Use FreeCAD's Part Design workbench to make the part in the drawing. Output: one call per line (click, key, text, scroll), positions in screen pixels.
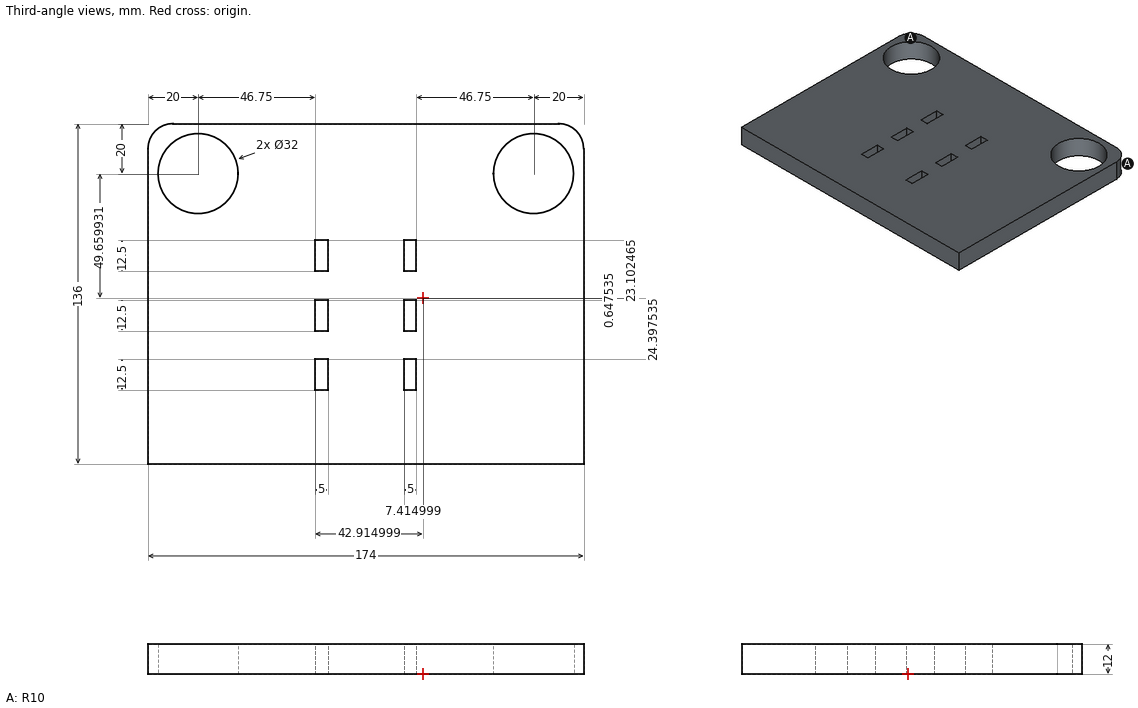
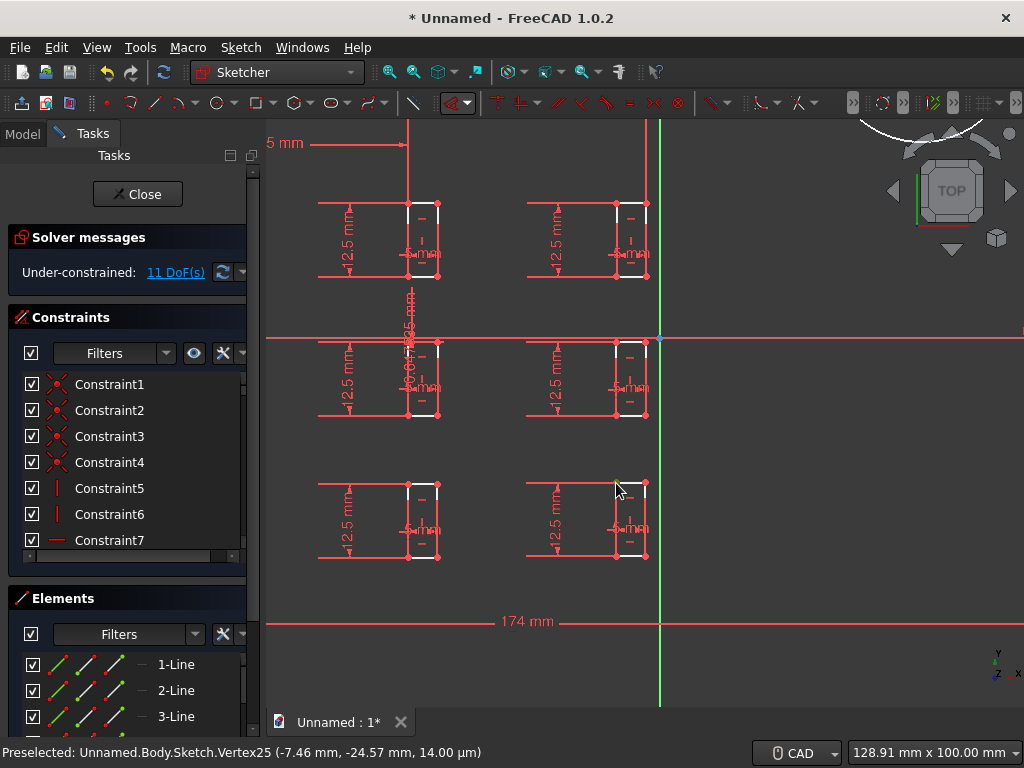
key(l)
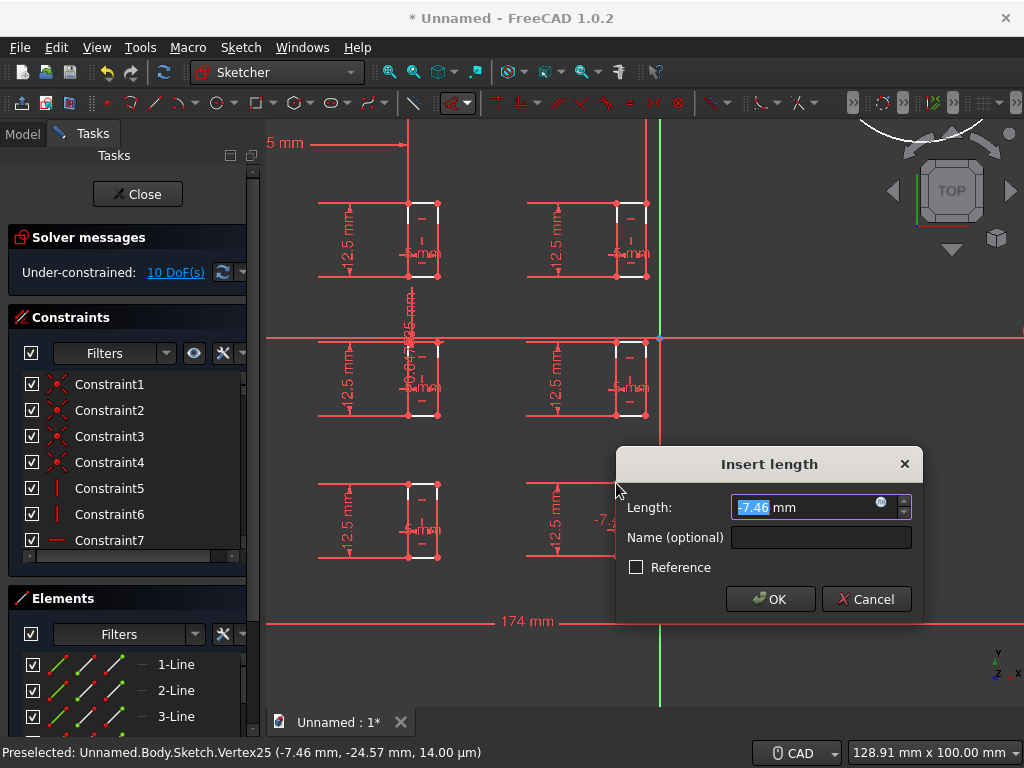
text(-7.414999)
key(Return)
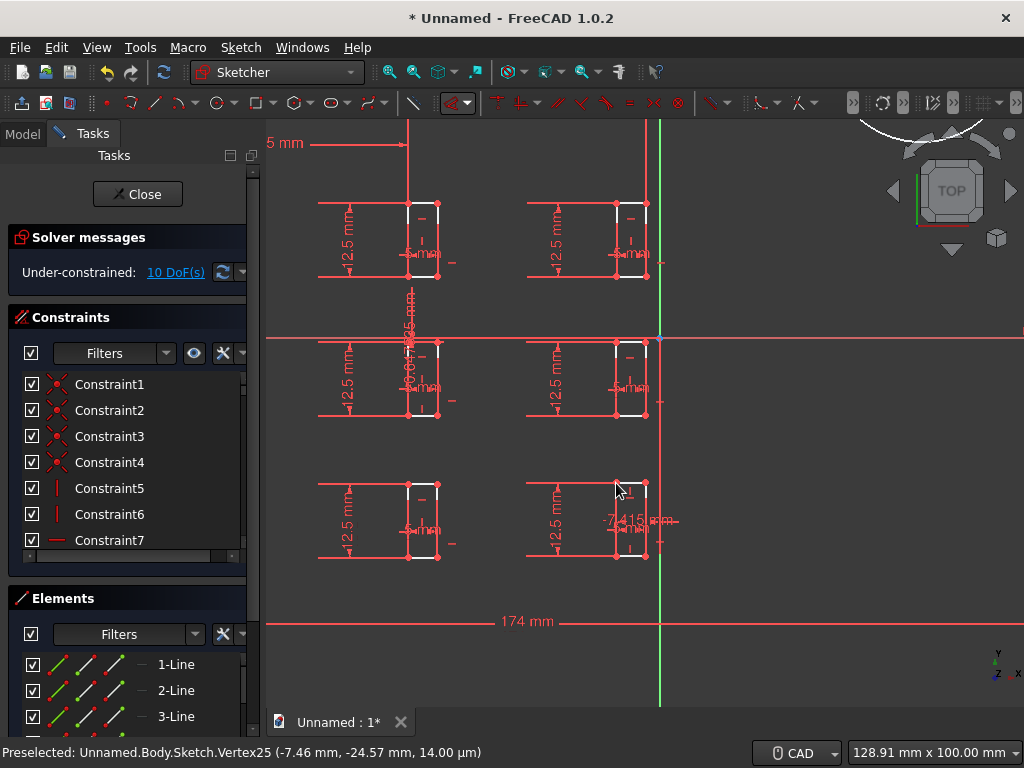
click(616, 342)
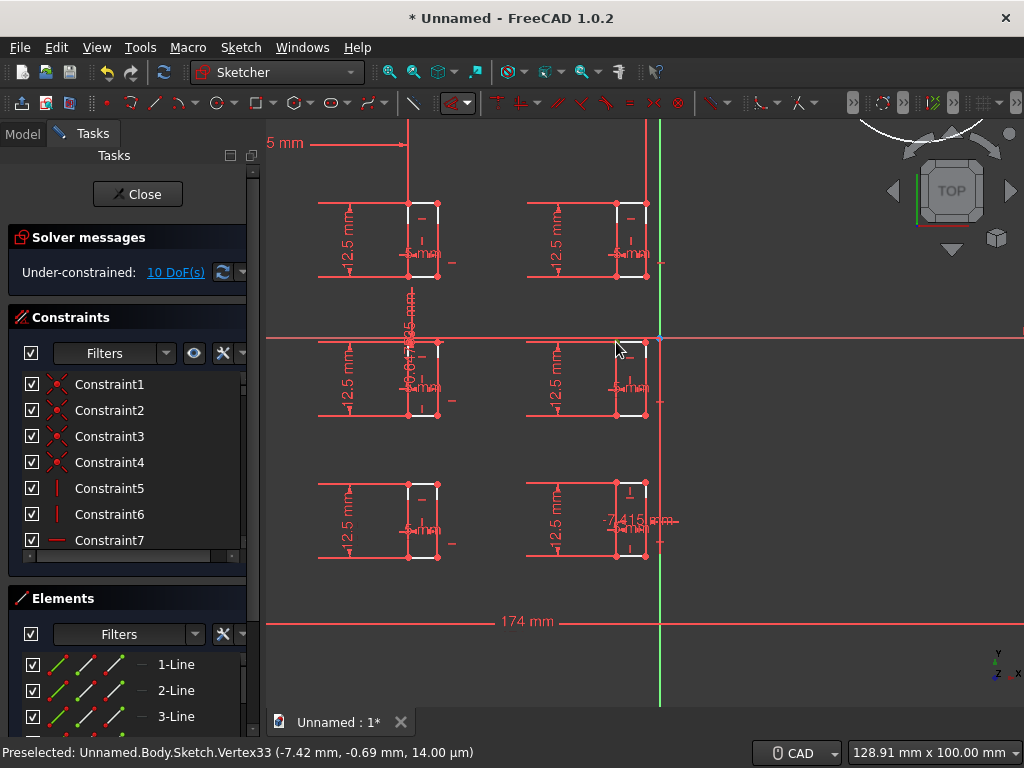
click(470, 104)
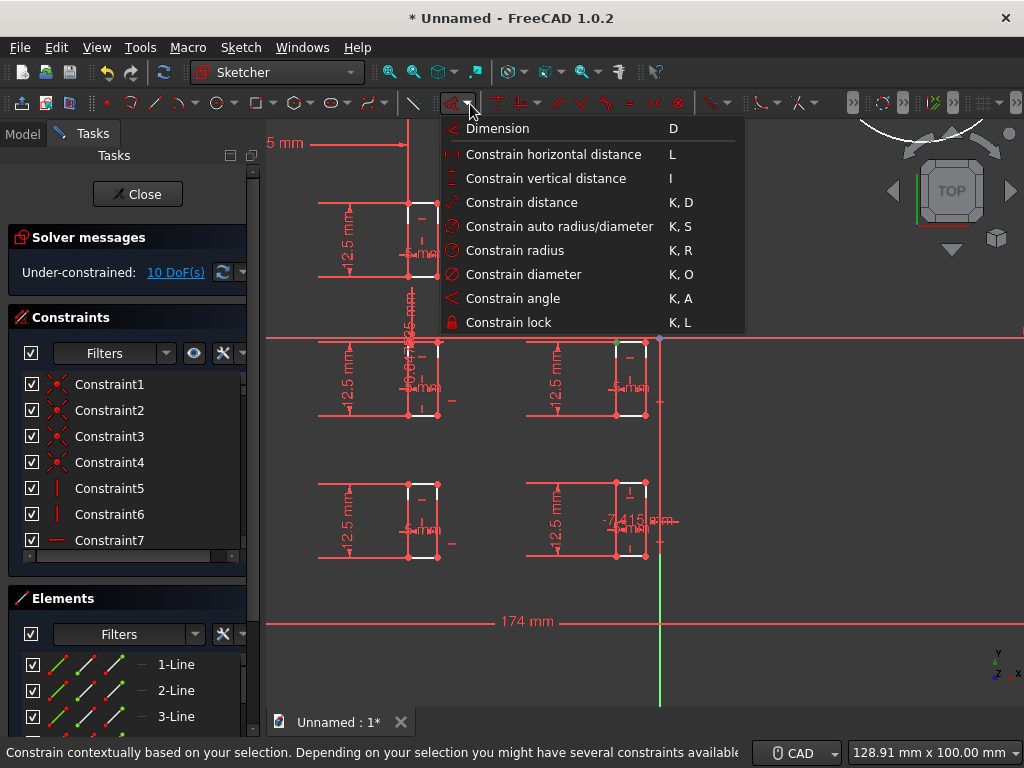
click(593, 154)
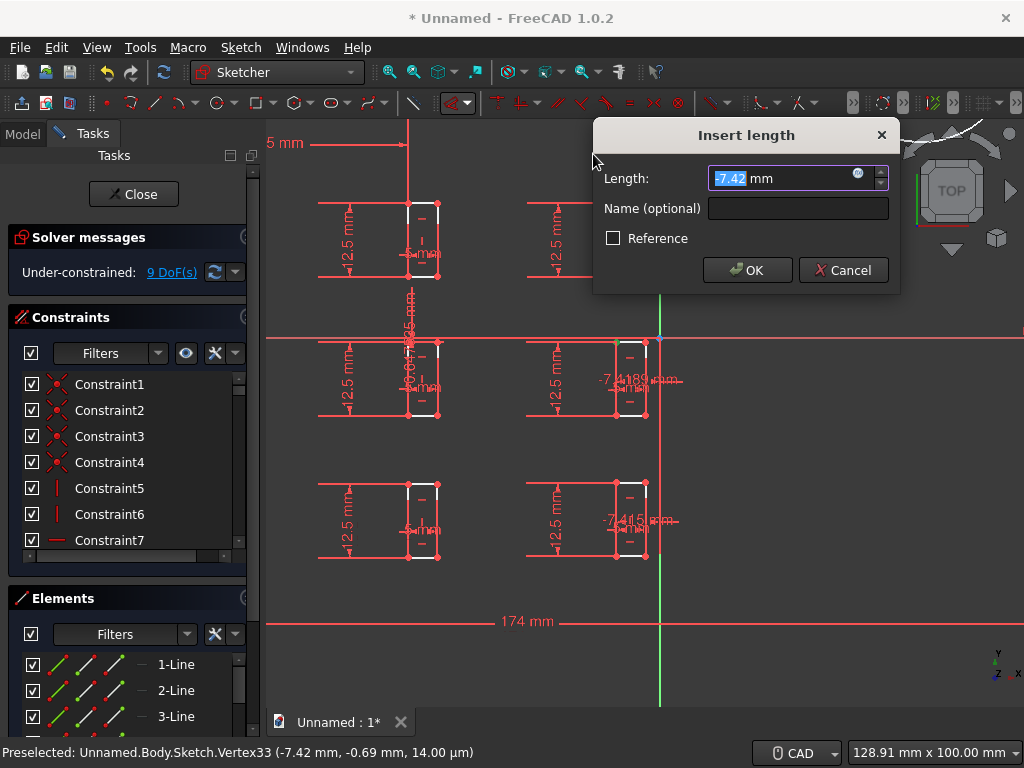
text(-7.414999)
key(Return)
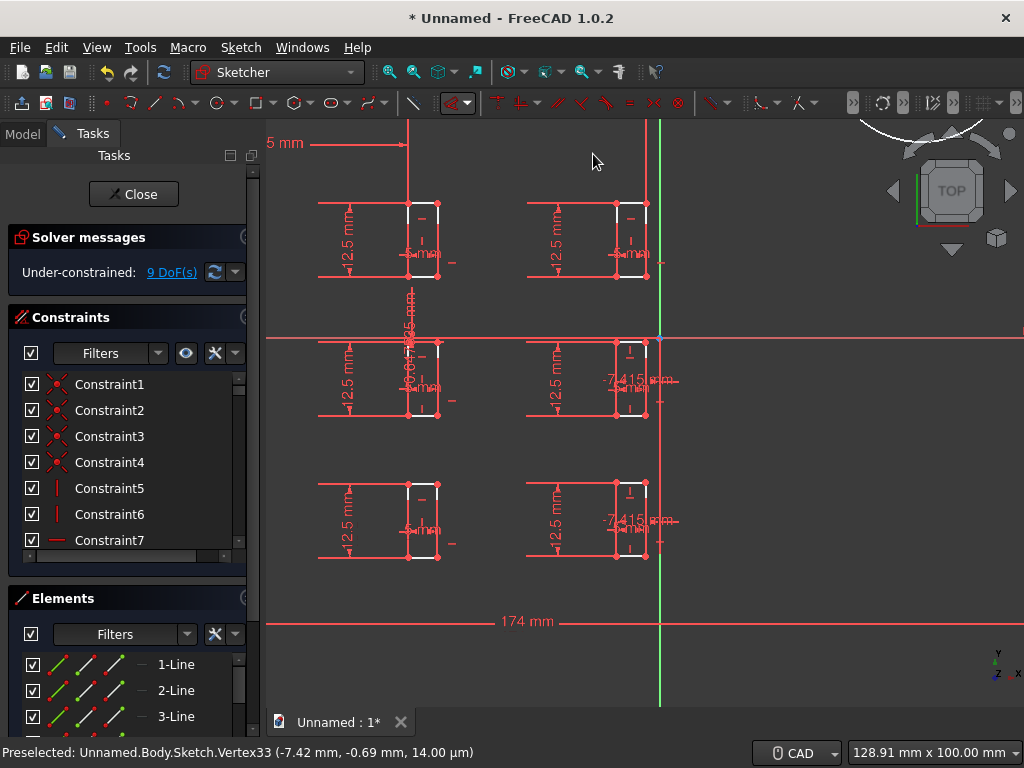
scroll(616, 342, up, 12)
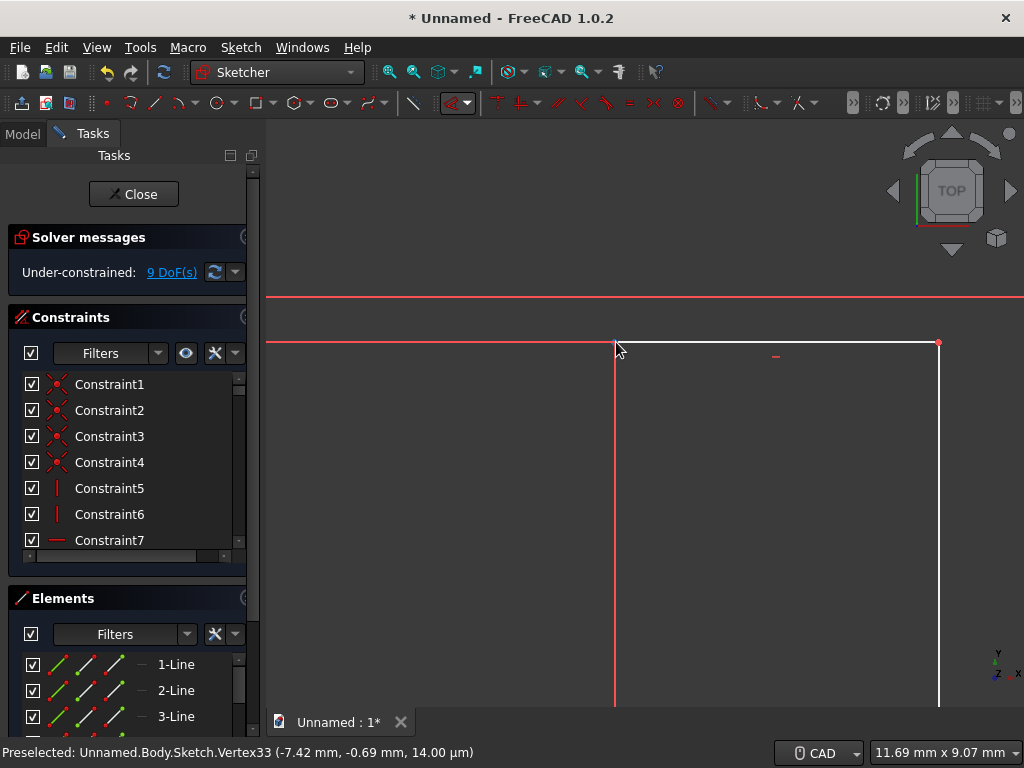
click(615, 342)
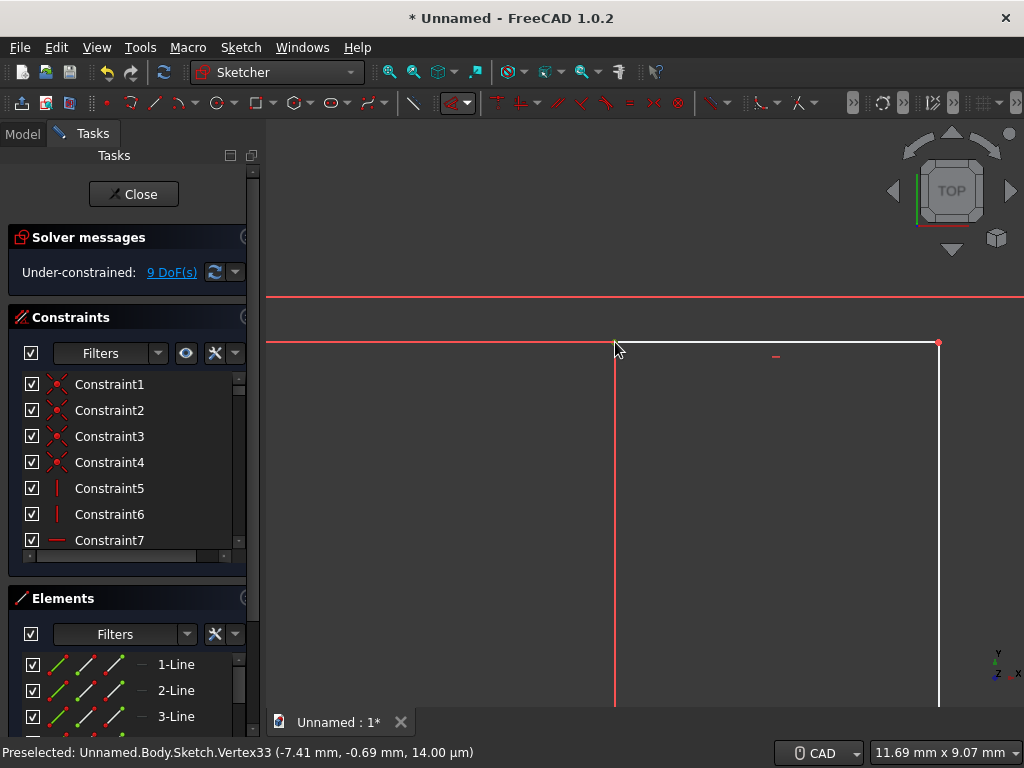
click(470, 104)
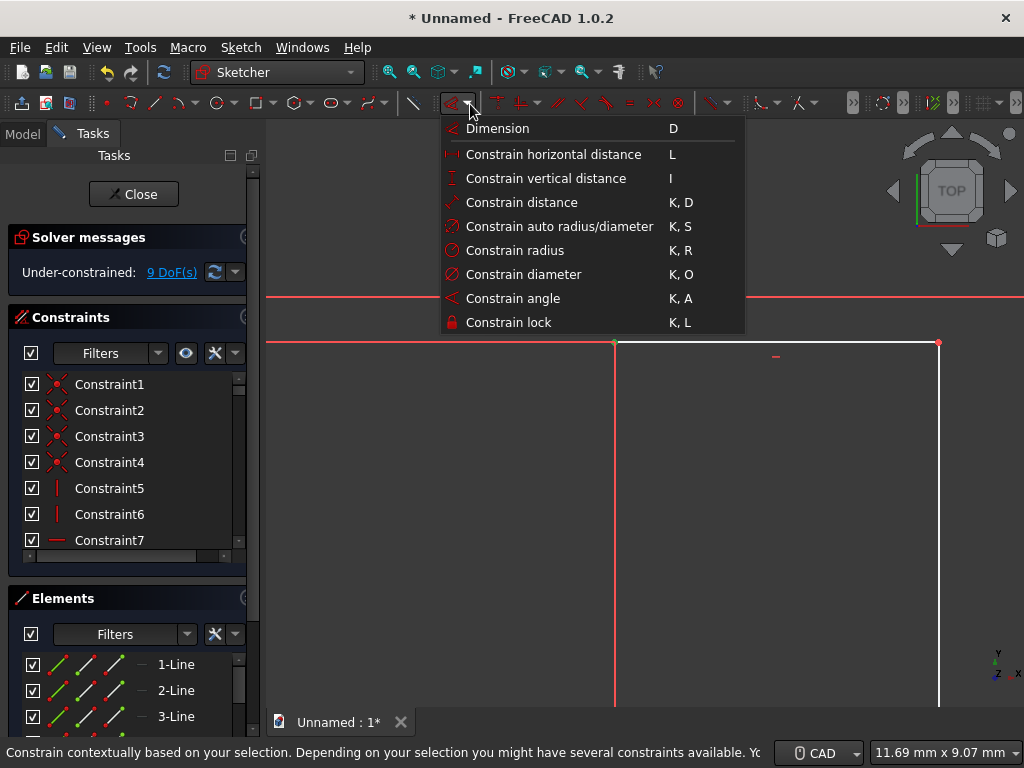
click(593, 178)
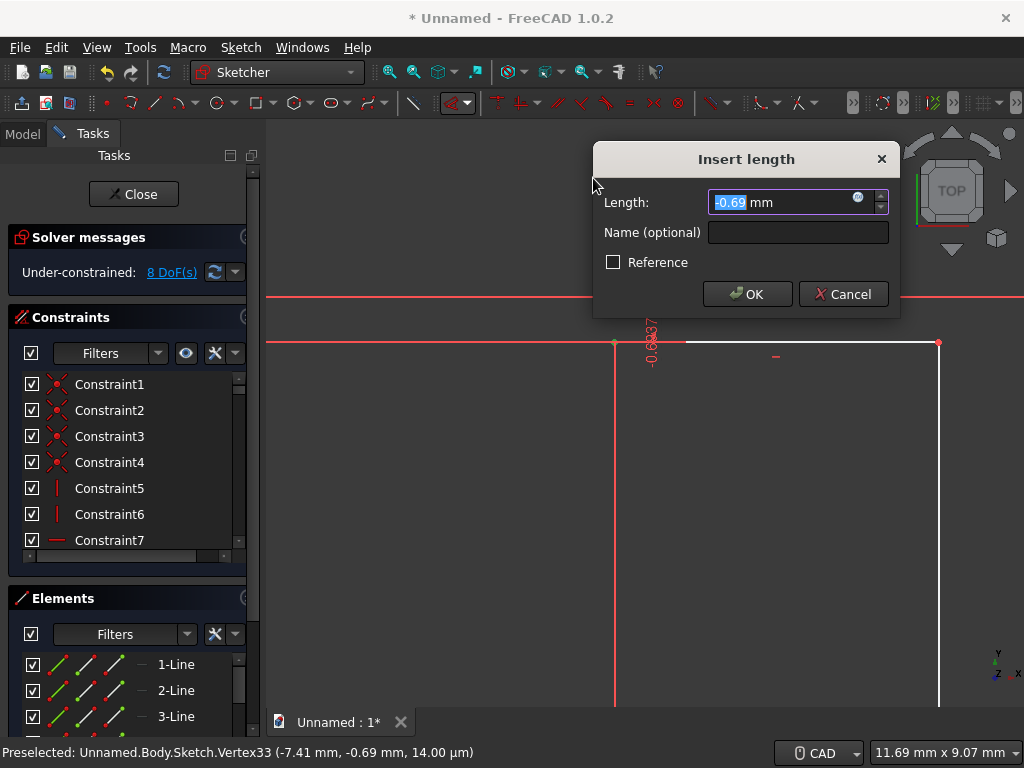
text(-0.647535)
key(Return)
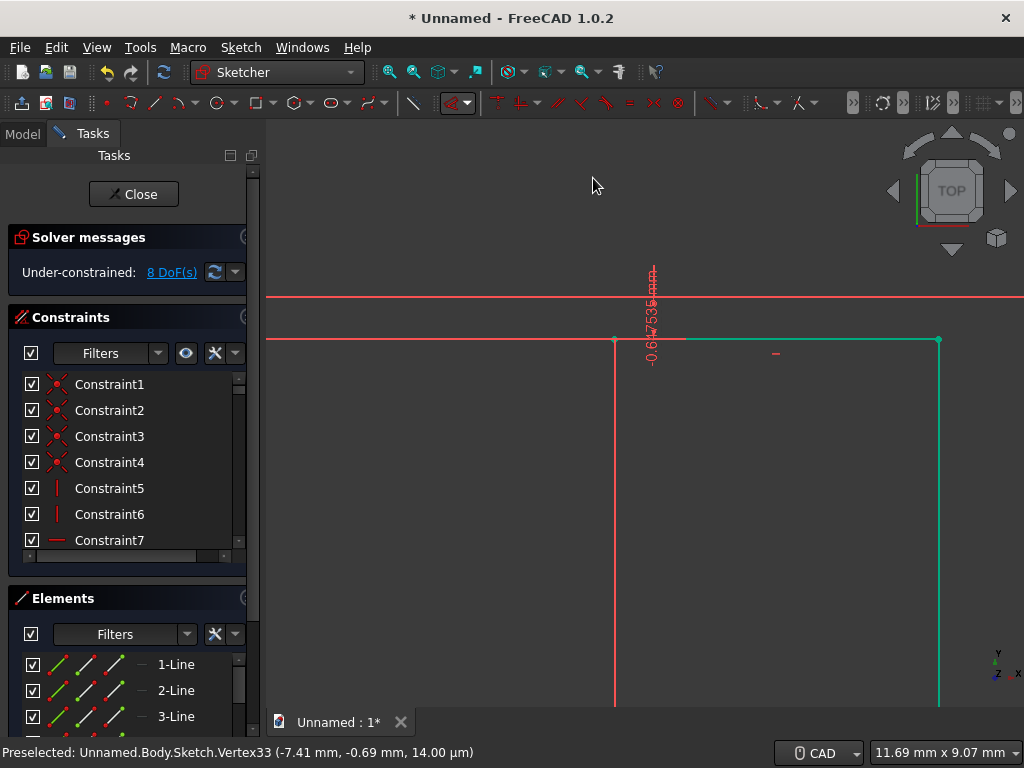
scroll(617, 422, down, 16)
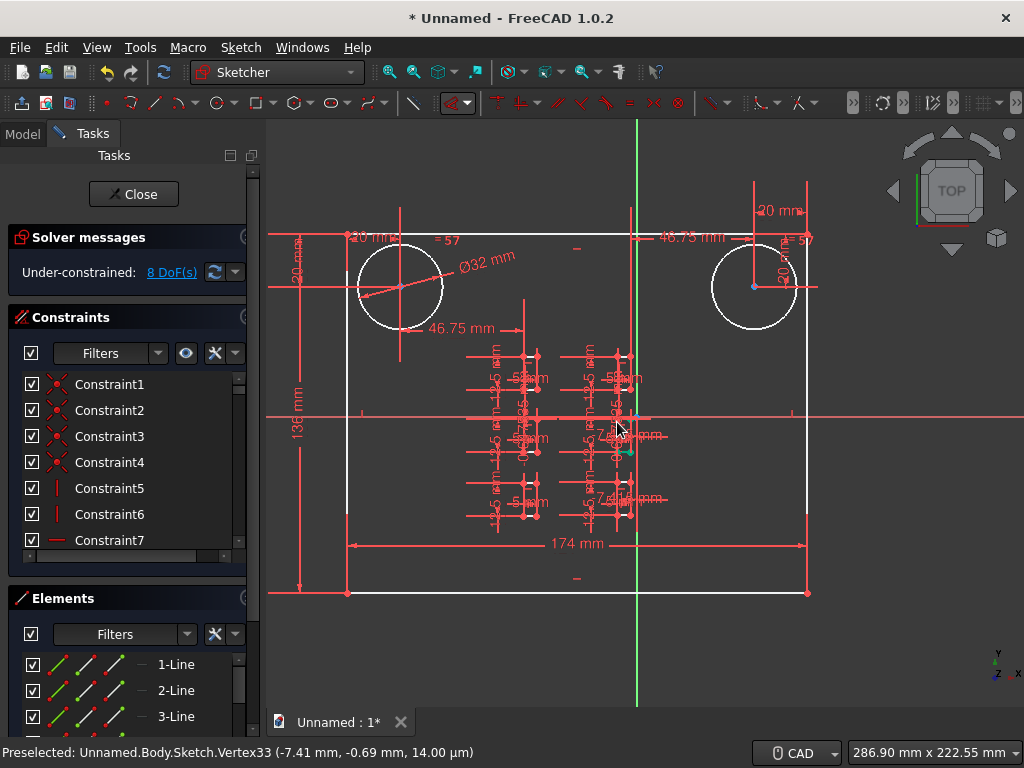
scroll(618, 357, up, 4)